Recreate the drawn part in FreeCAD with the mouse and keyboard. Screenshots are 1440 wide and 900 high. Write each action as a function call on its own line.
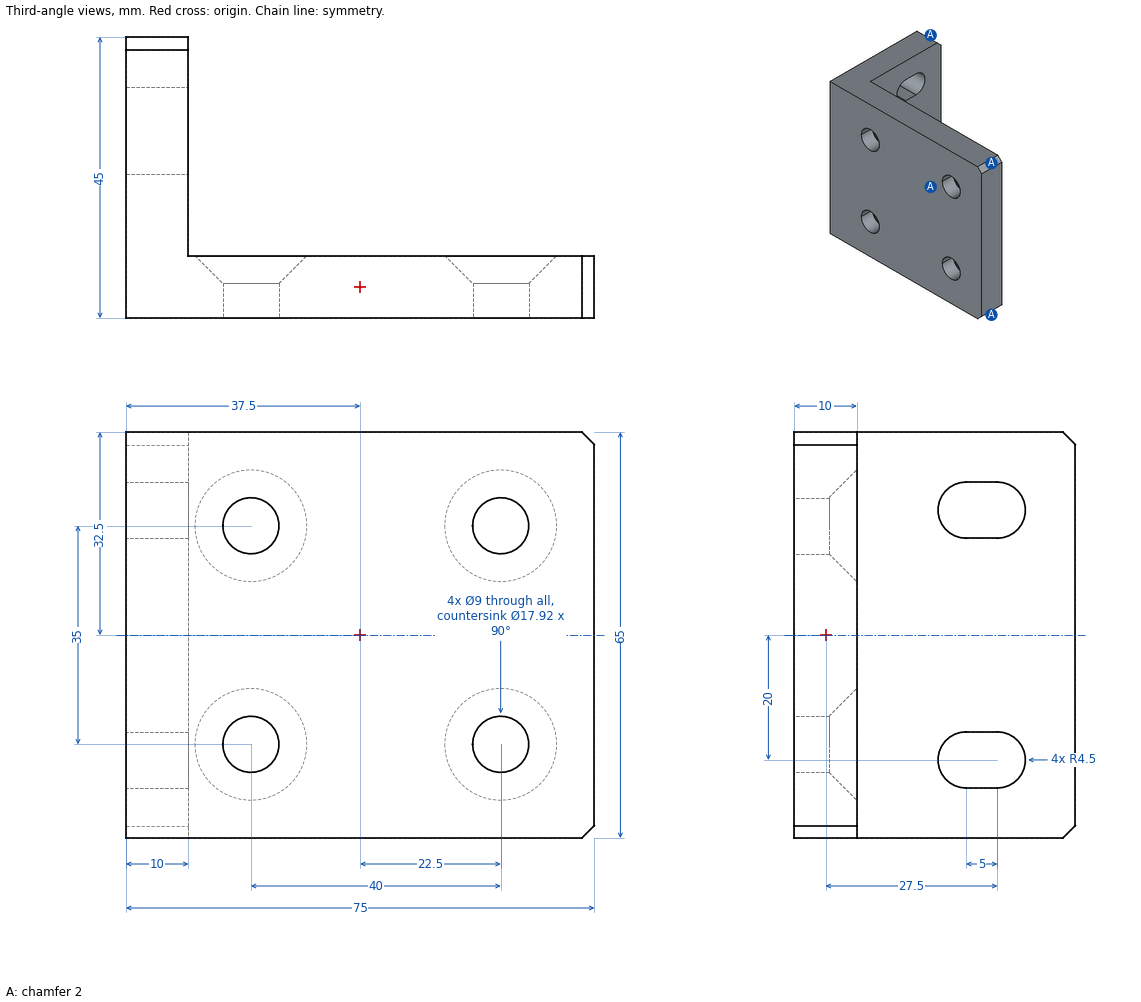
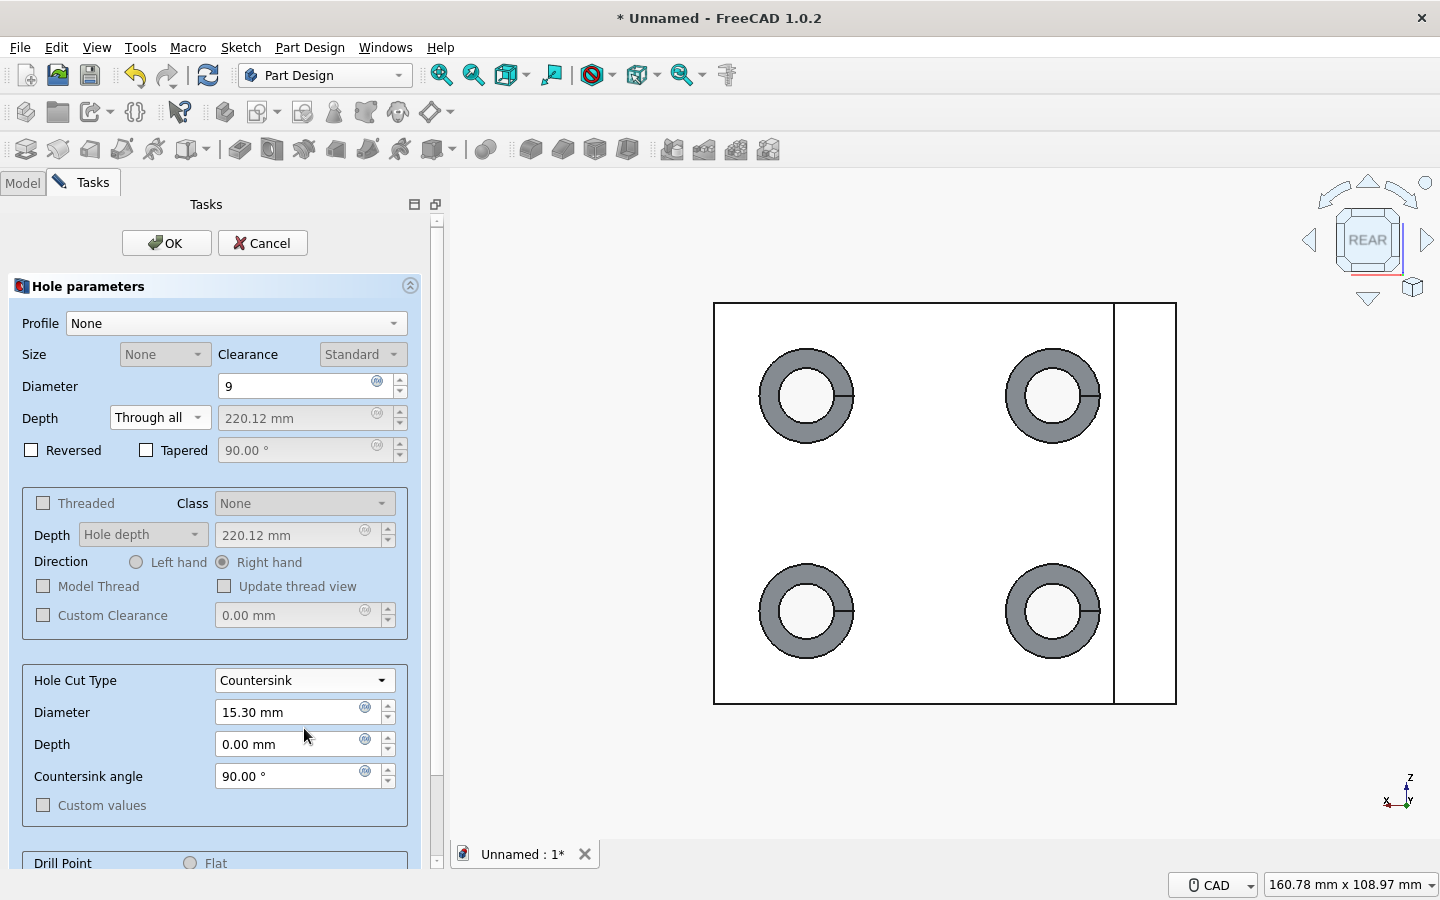
triple_click(298, 712)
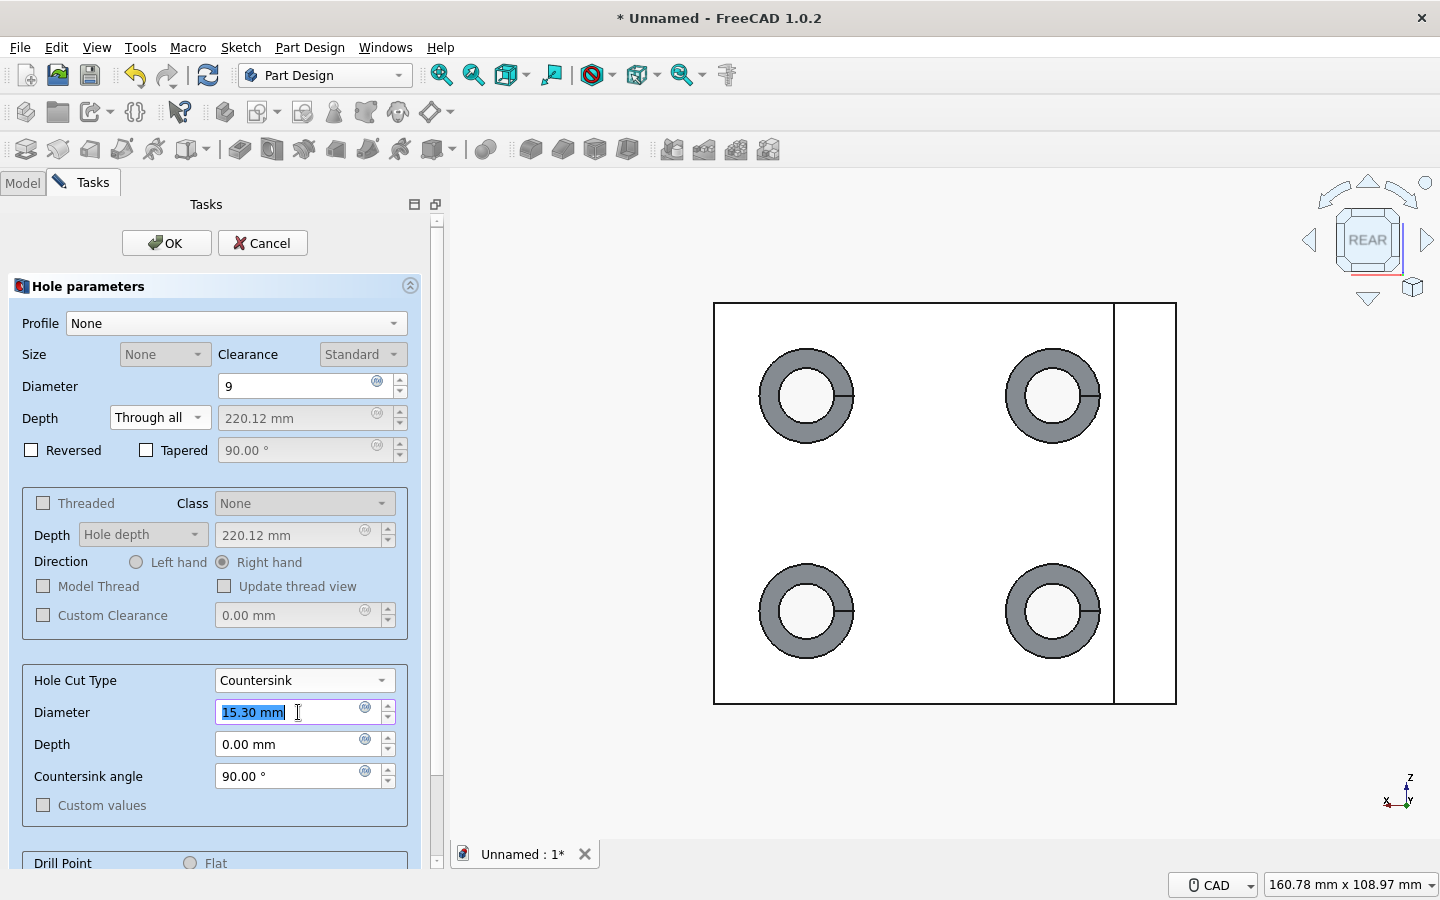
text(17.92)
key(Tab)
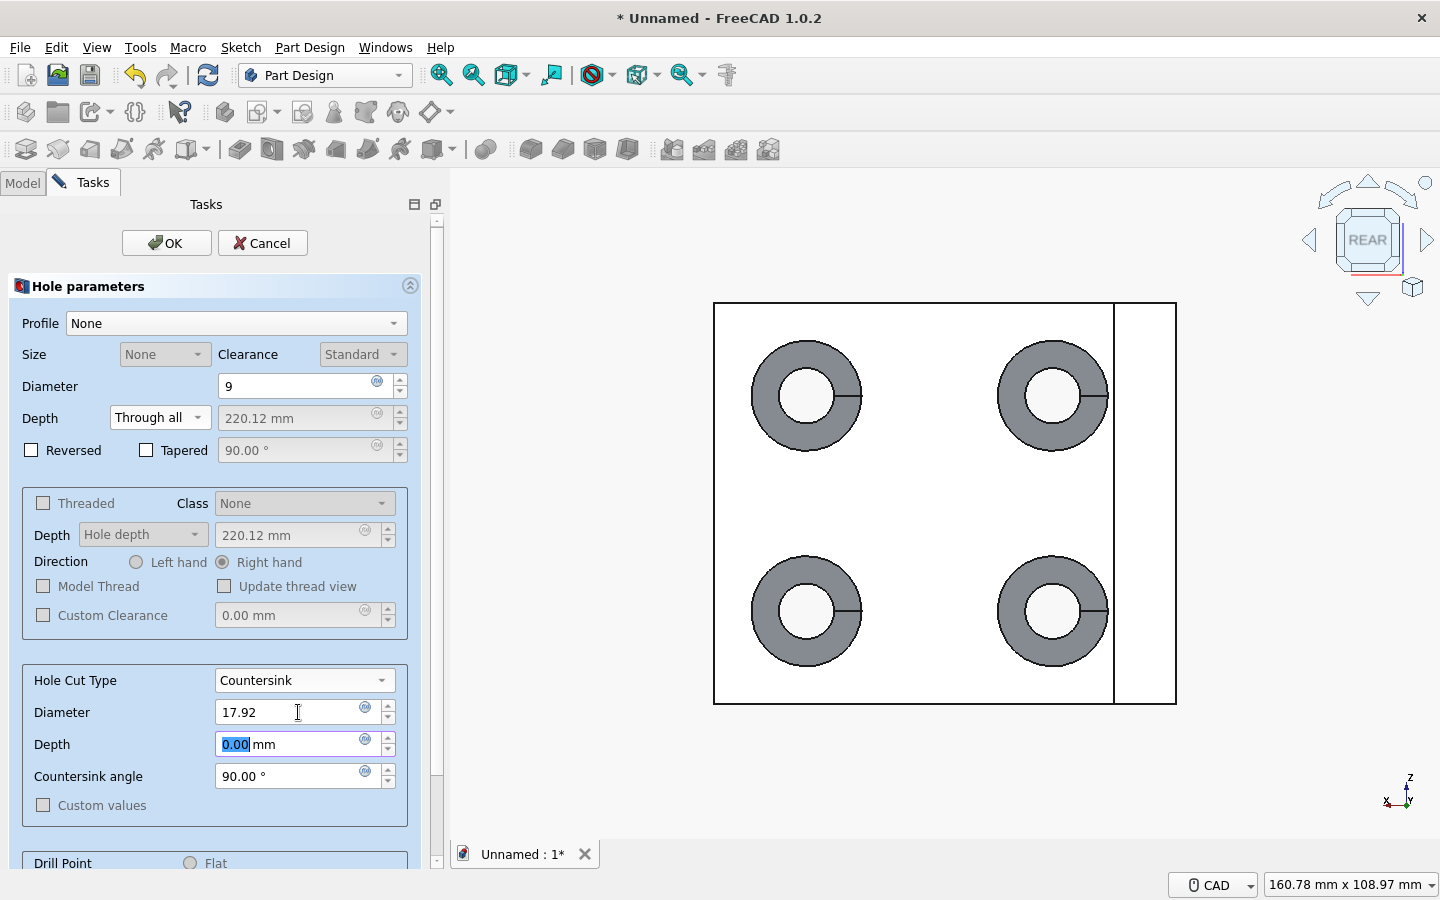
click(167, 243)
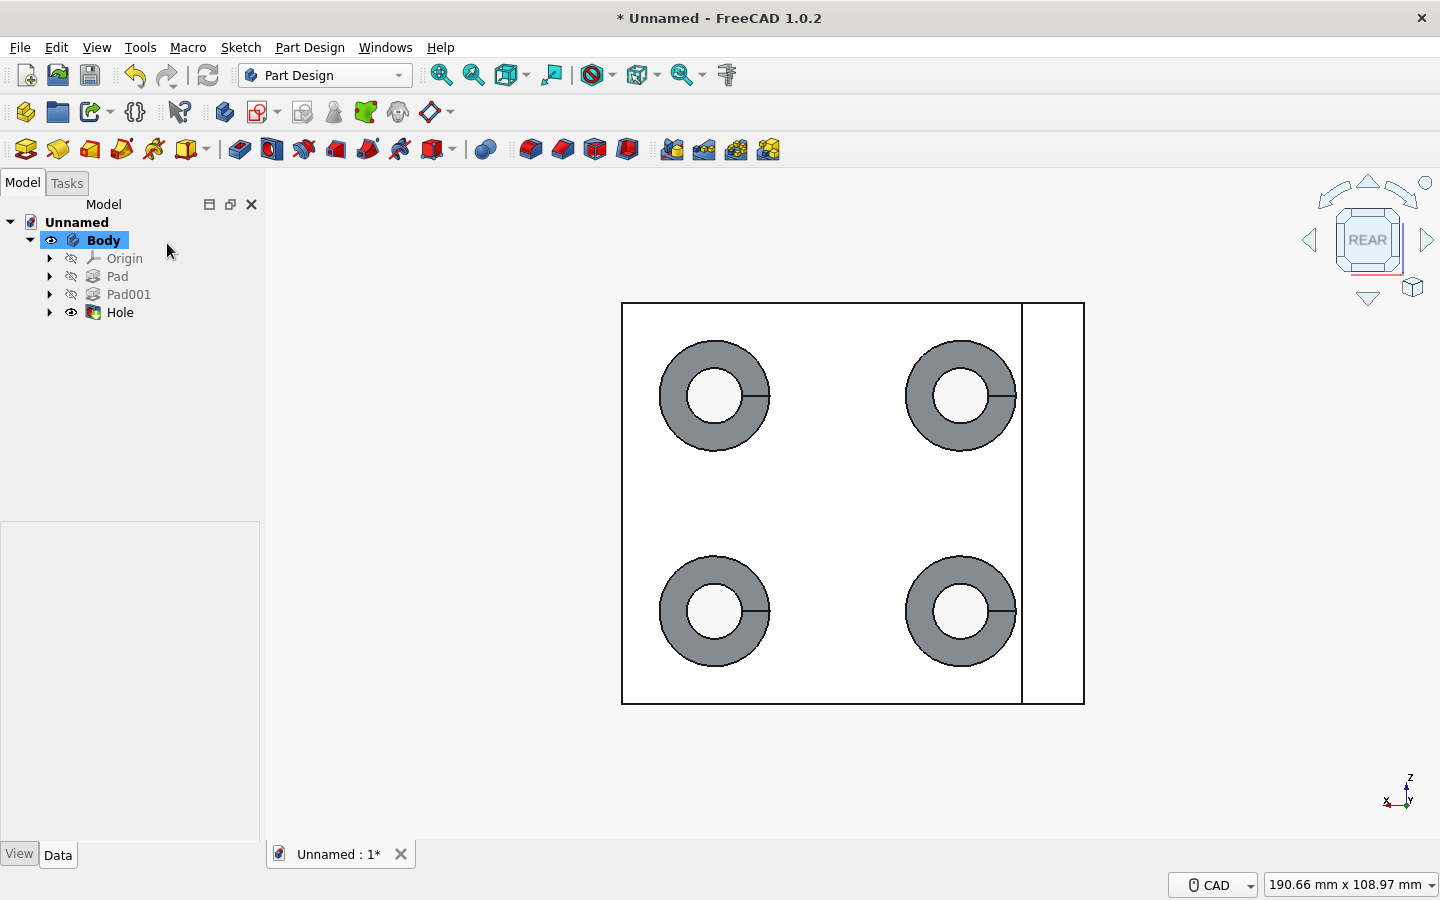
key(0)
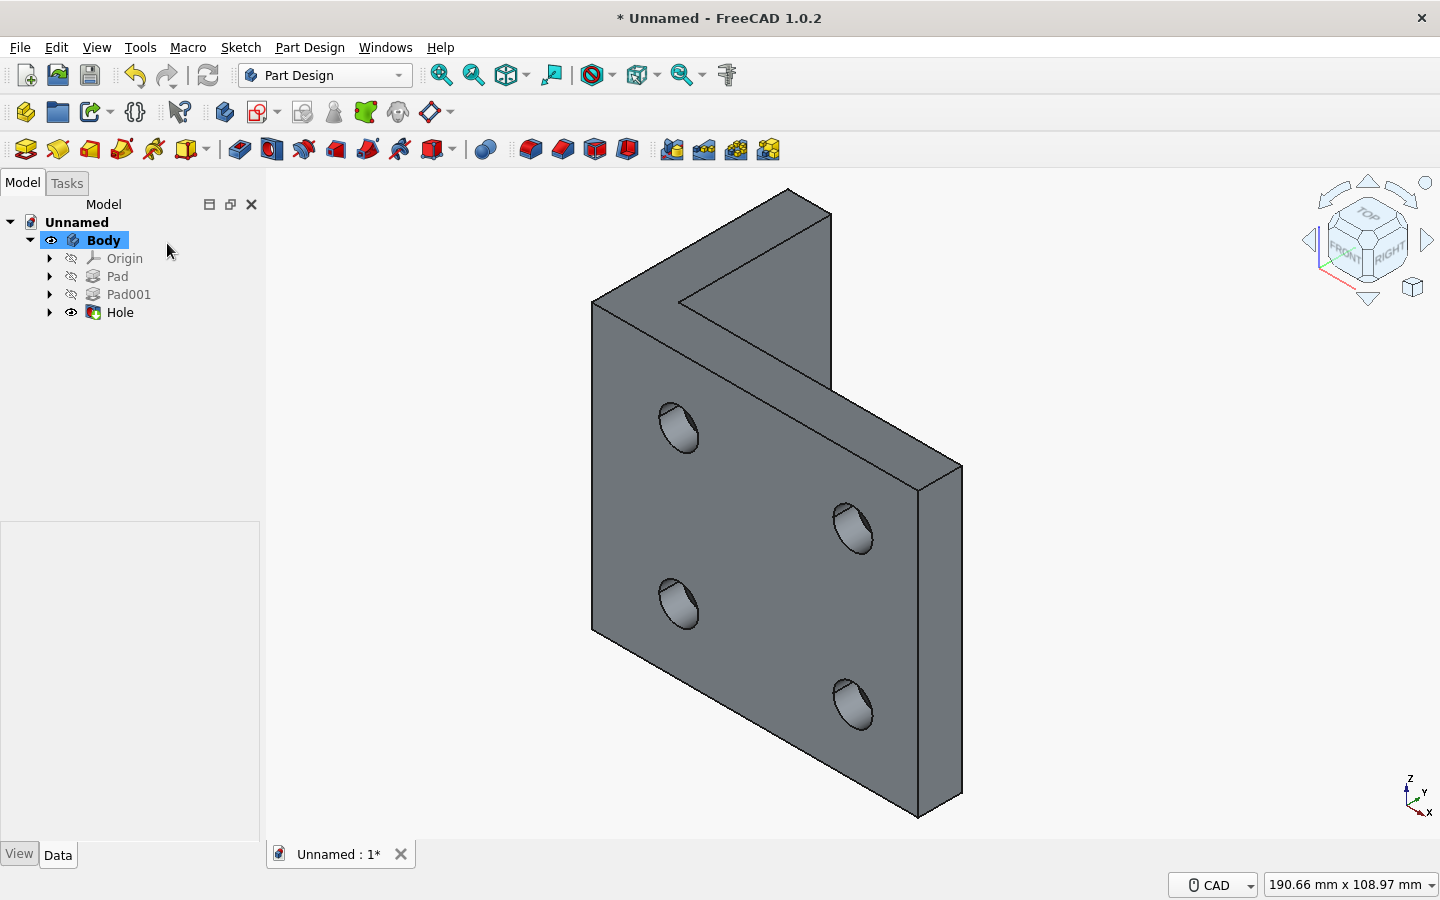
click(755, 327)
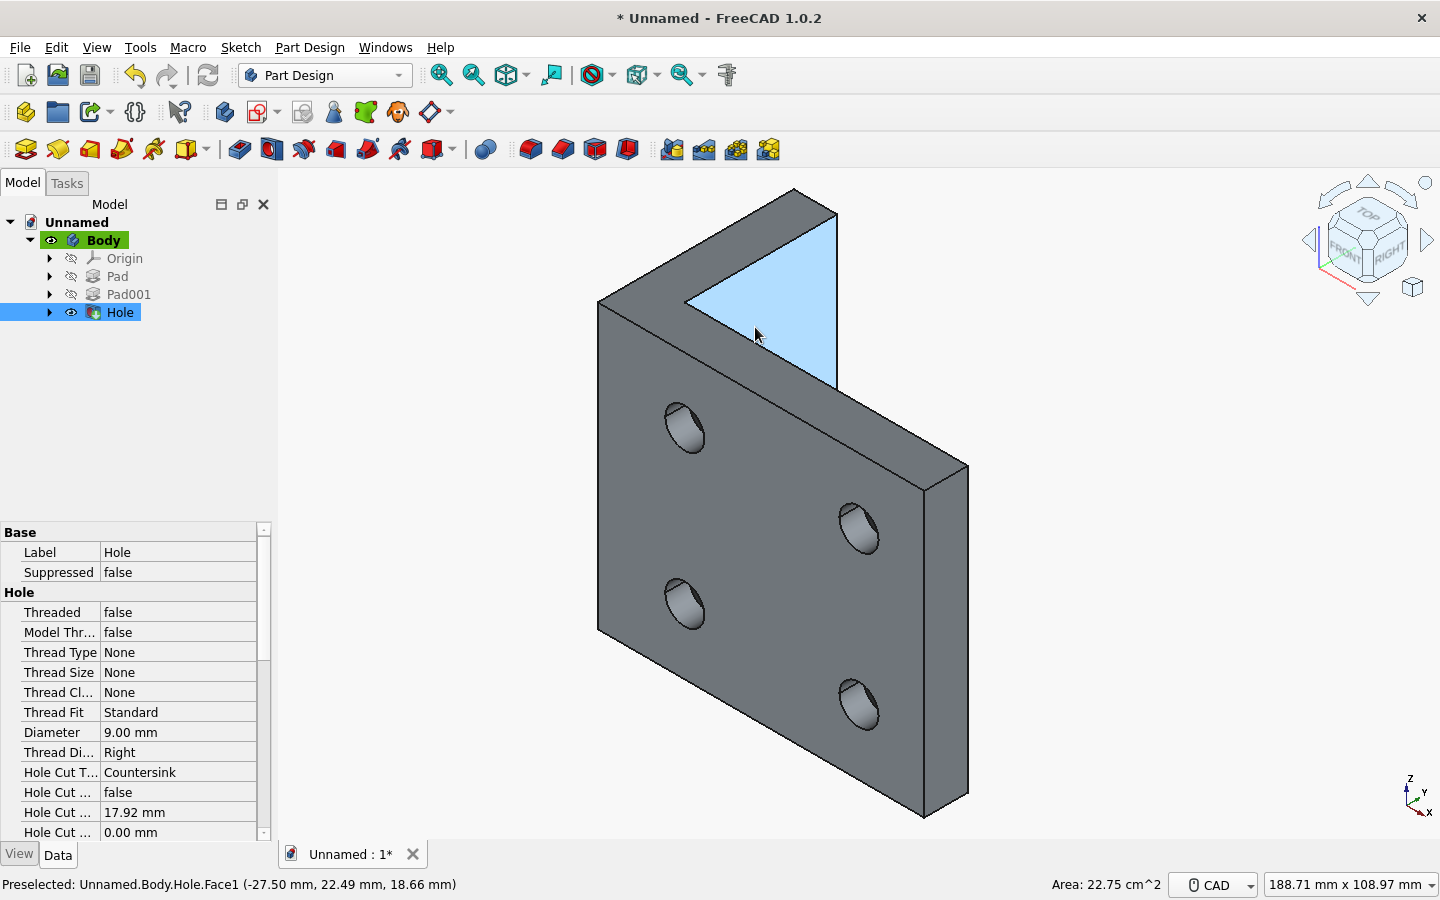
click(258, 112)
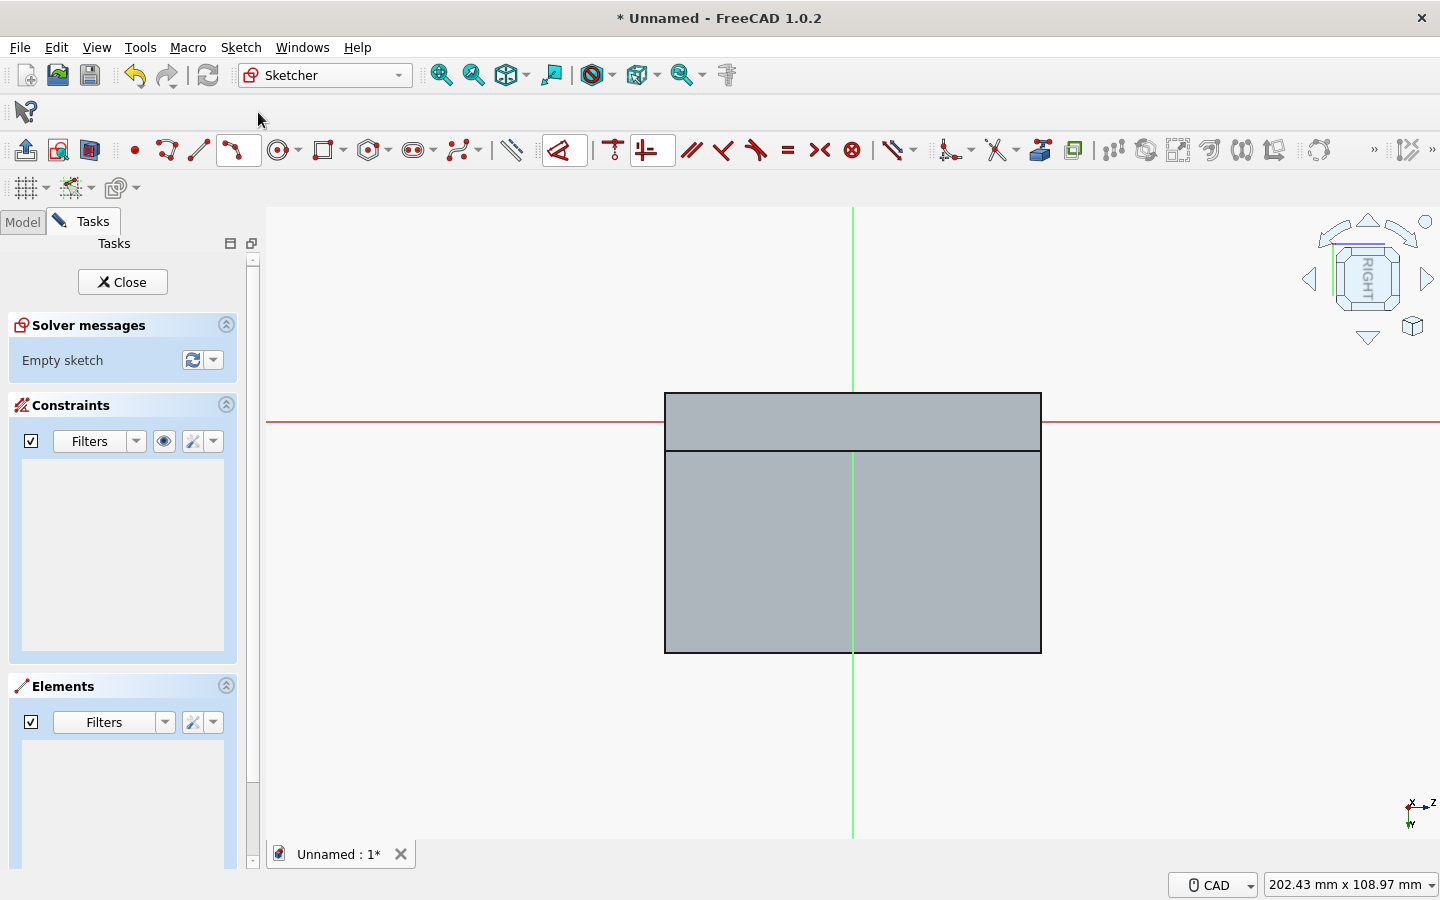
key(q)
key(s)